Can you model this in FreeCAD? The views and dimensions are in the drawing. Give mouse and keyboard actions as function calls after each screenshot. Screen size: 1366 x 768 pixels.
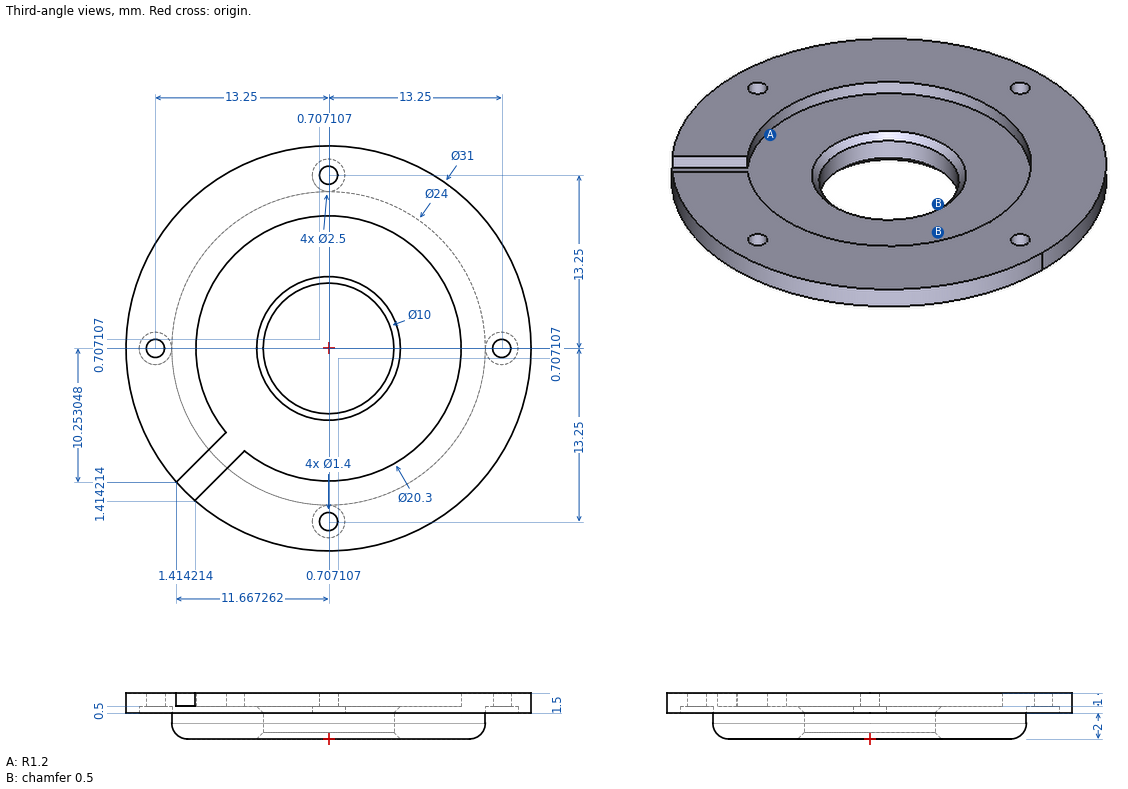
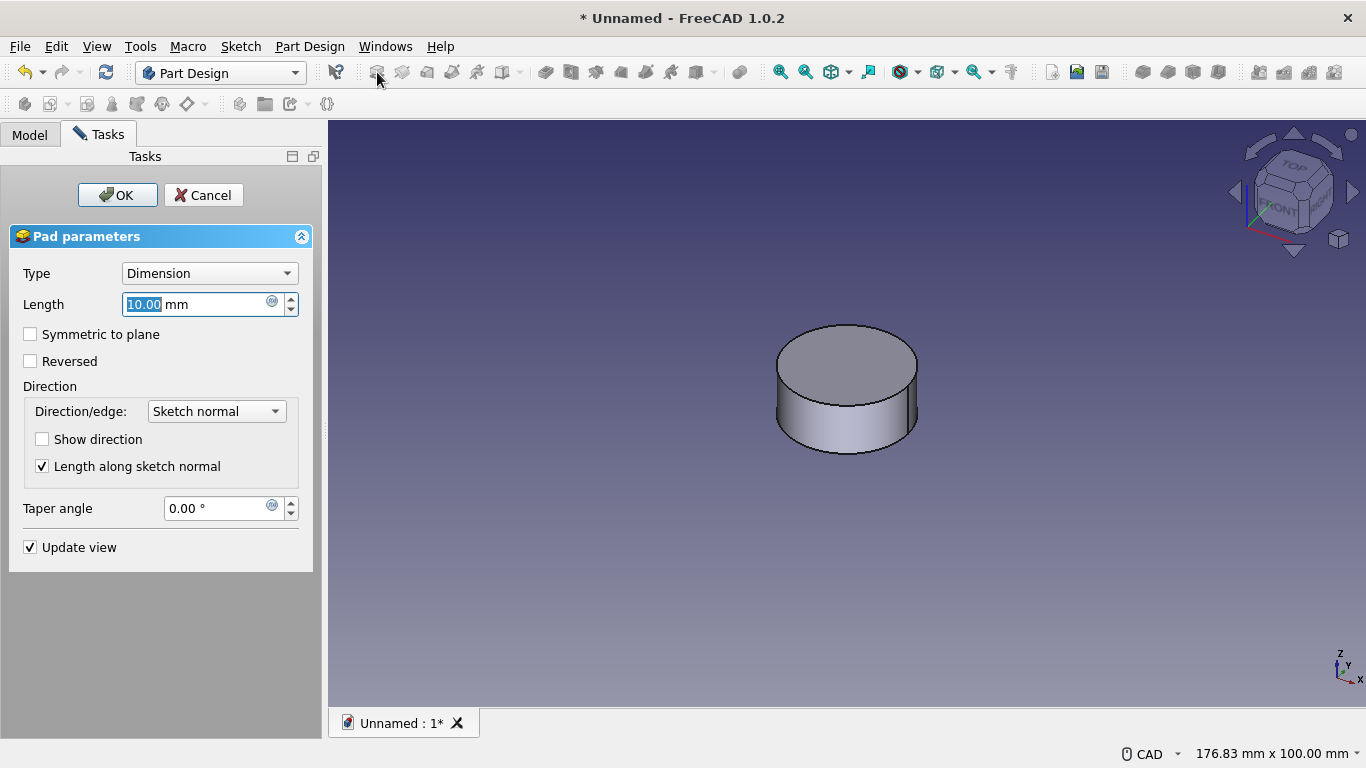
text(2)
key(Tab)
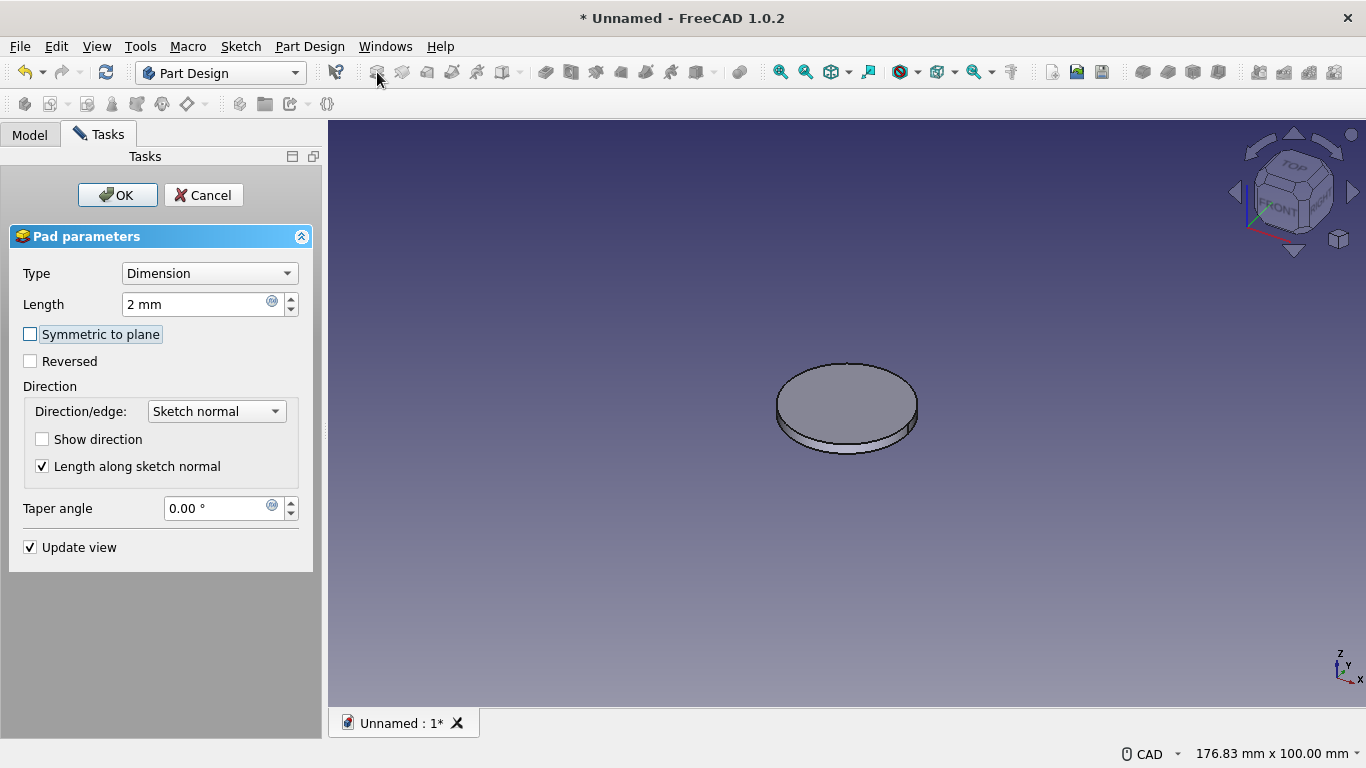
click(118, 195)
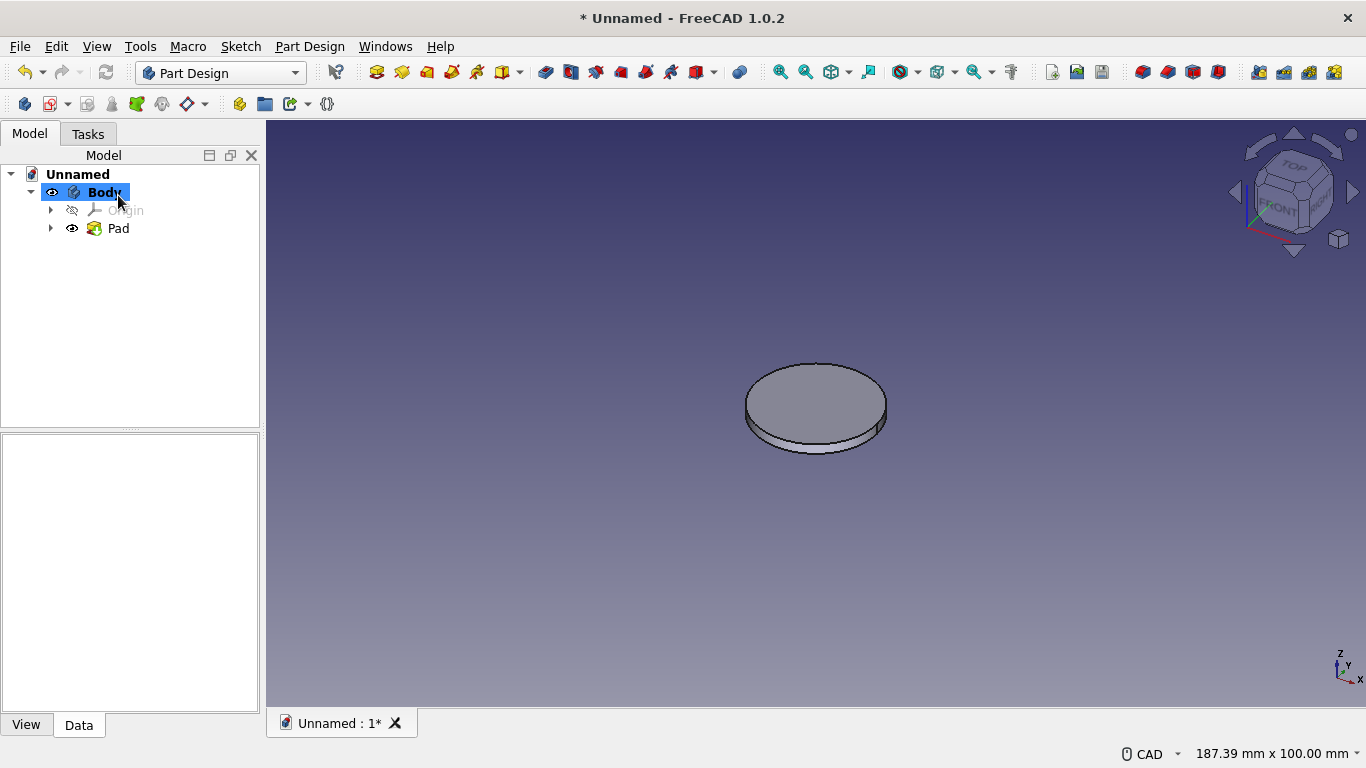
click(781, 72)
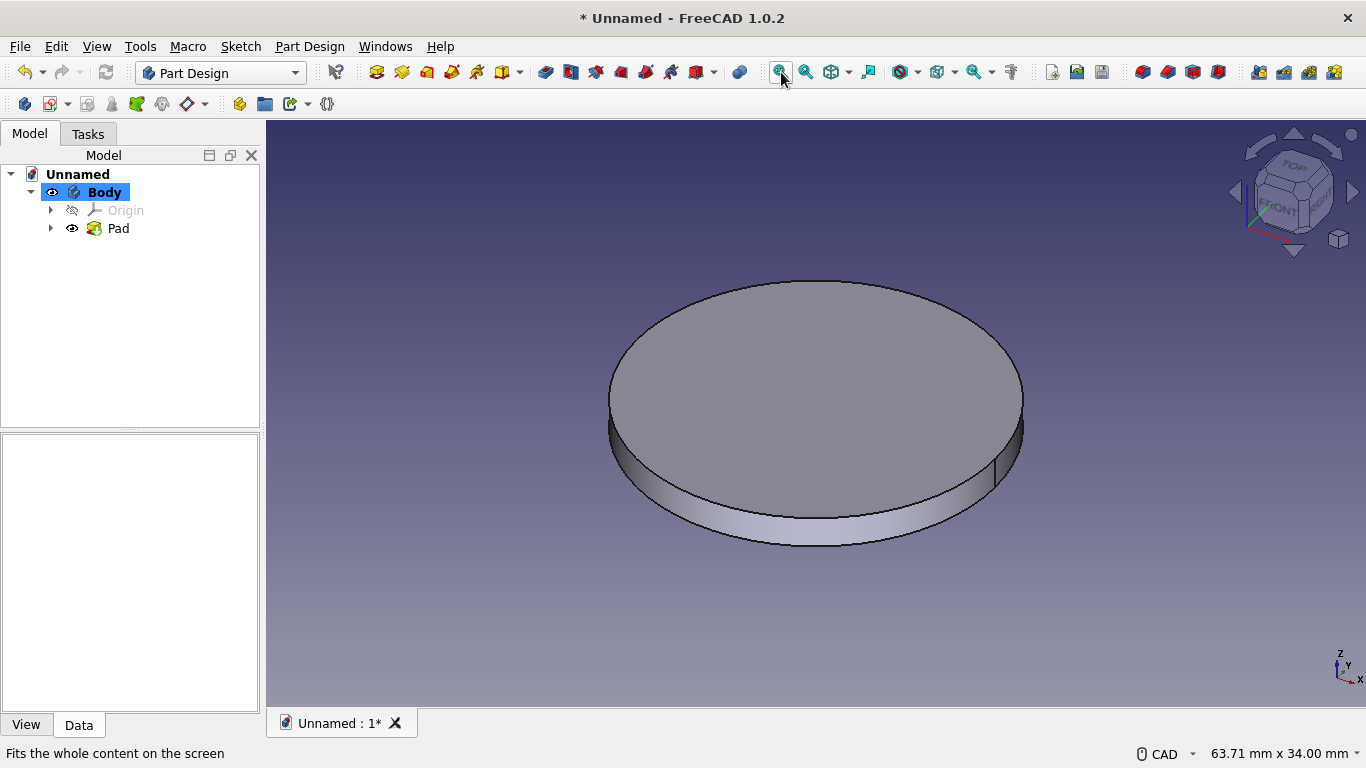
click(816, 398)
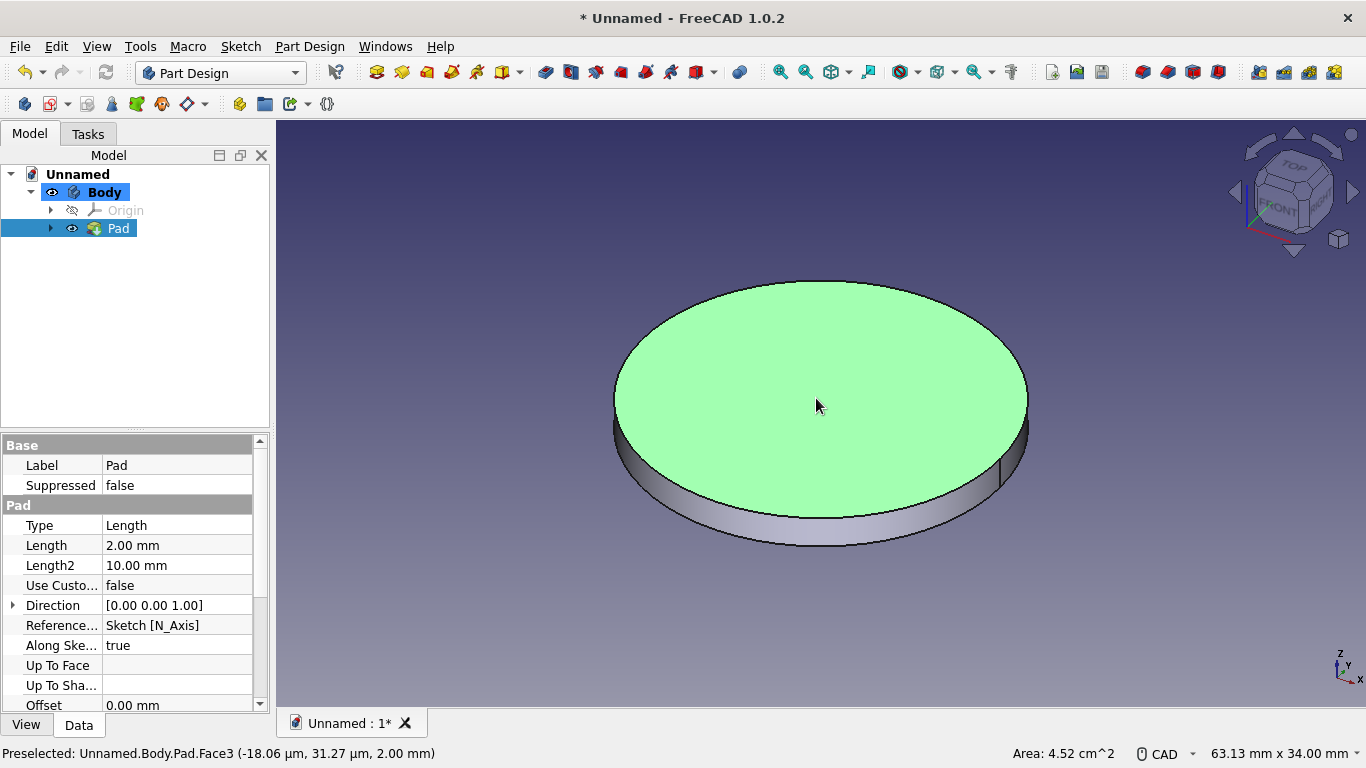
click(50, 104)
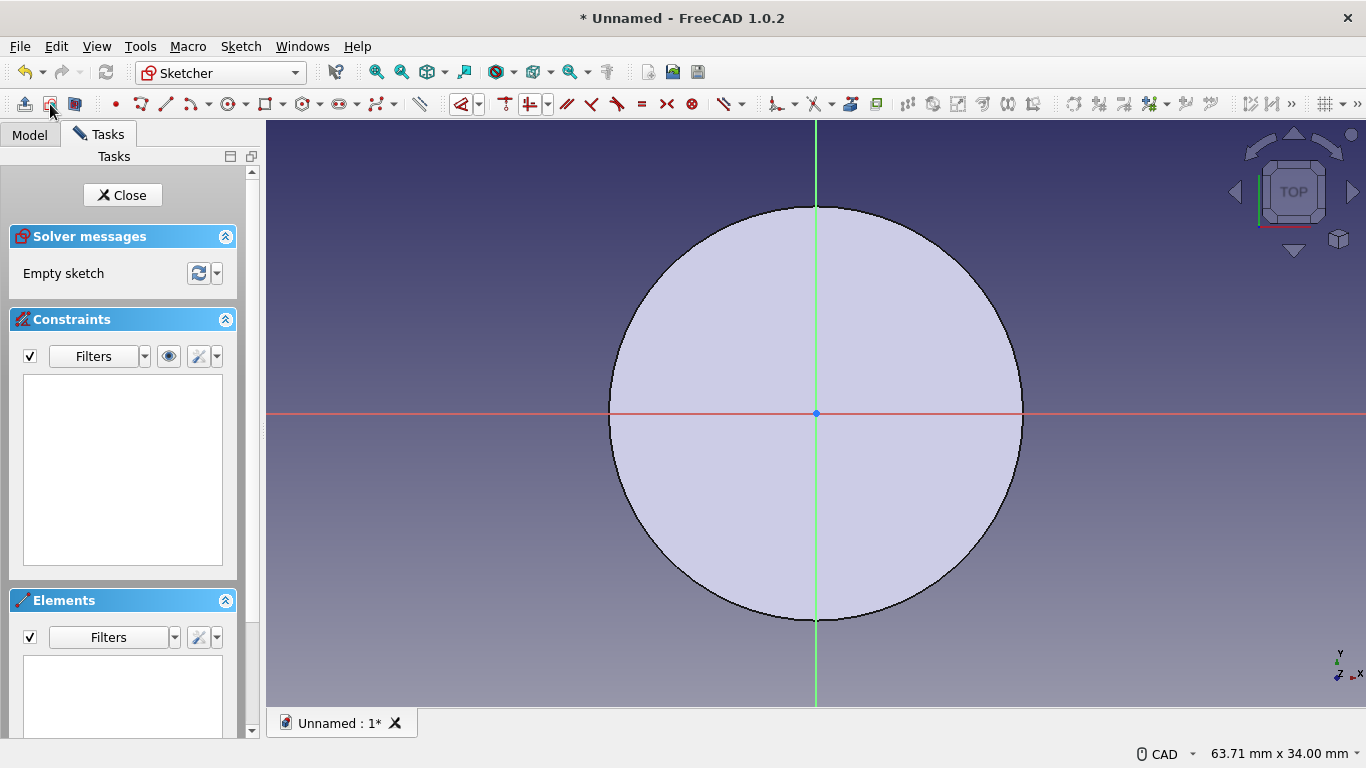
scroll(608, 414, down, 2)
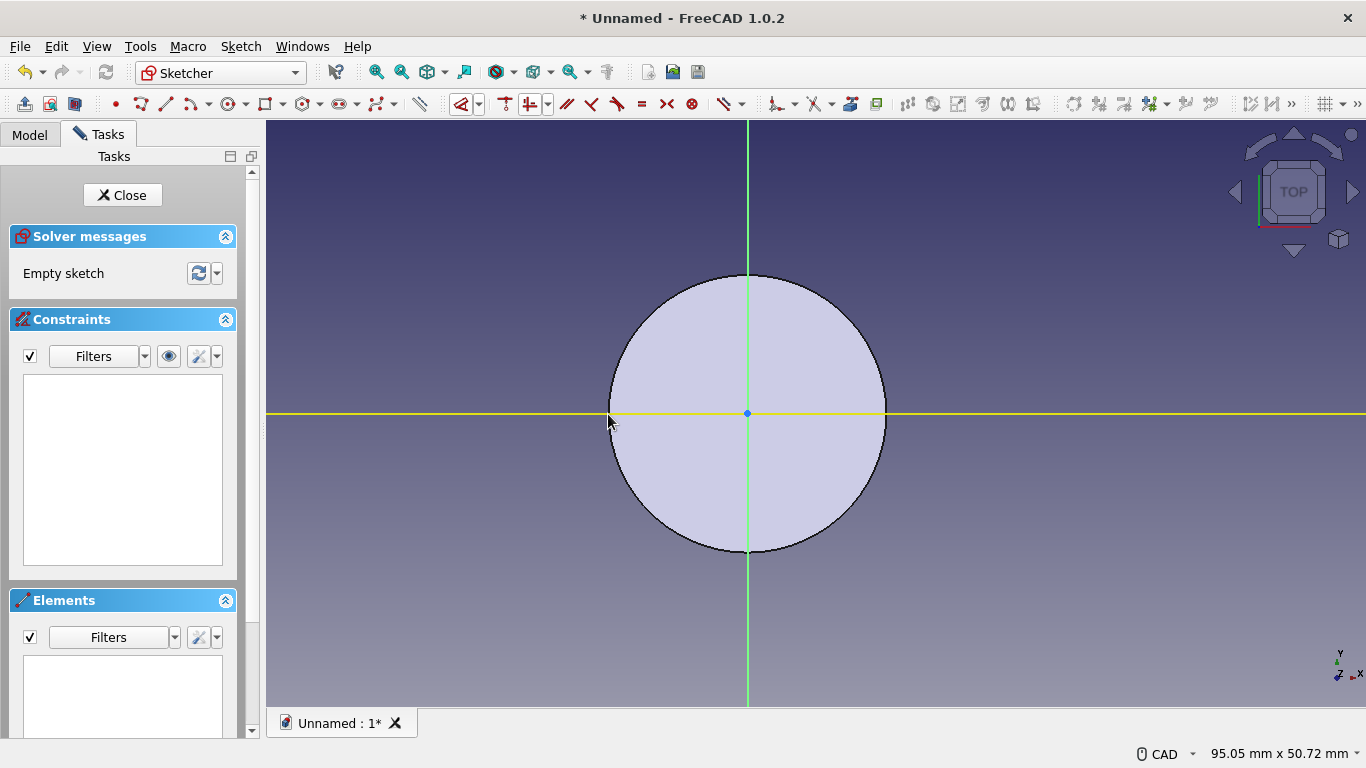
click(228, 104)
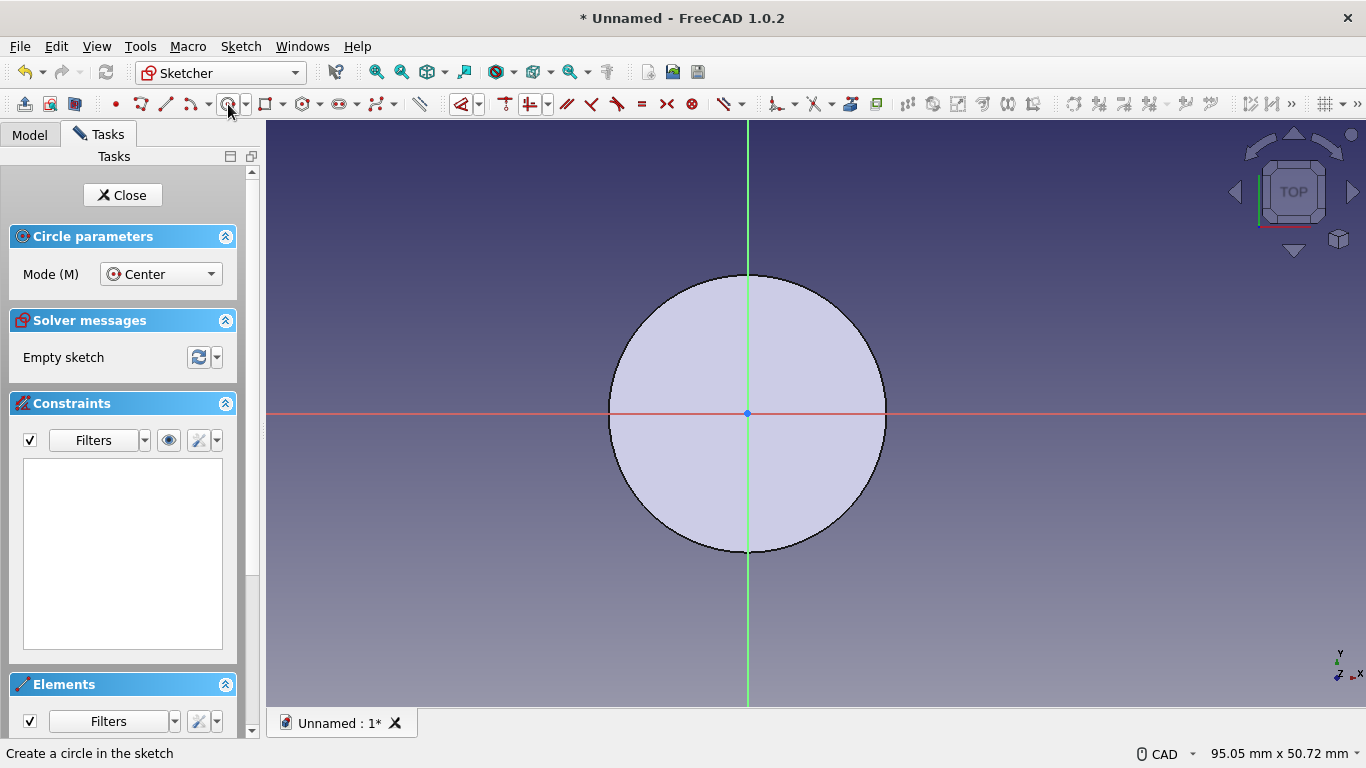
click(748, 414)
move(874, 287)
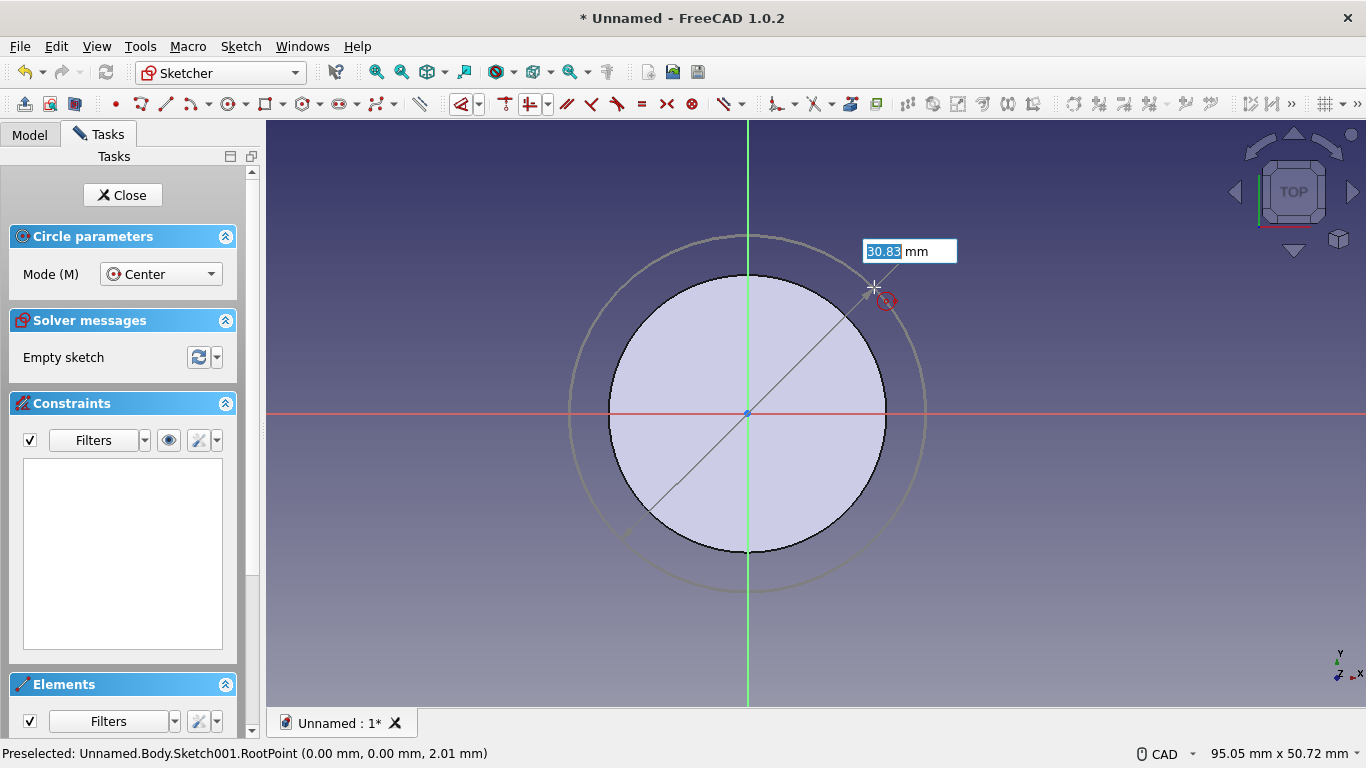
text(31)
key(Return)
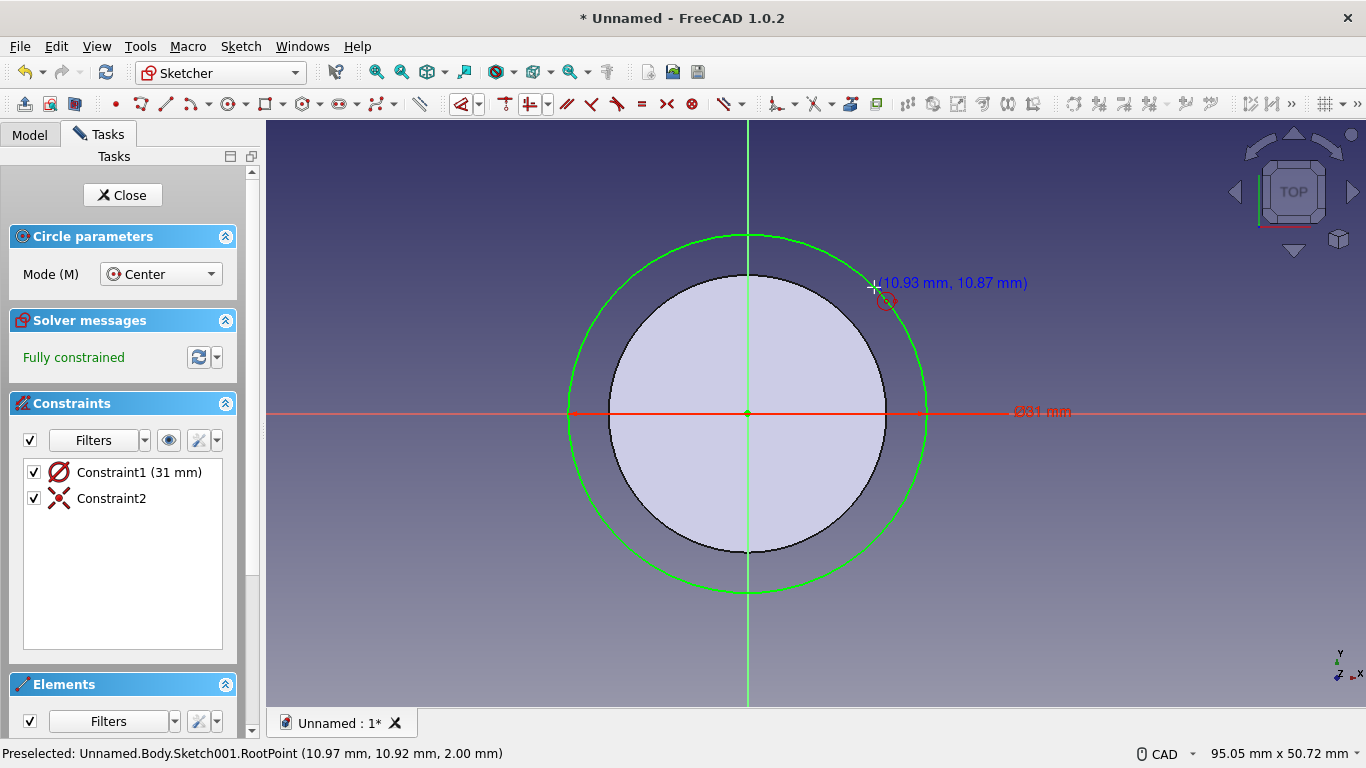
scroll(748, 567, up, 6)